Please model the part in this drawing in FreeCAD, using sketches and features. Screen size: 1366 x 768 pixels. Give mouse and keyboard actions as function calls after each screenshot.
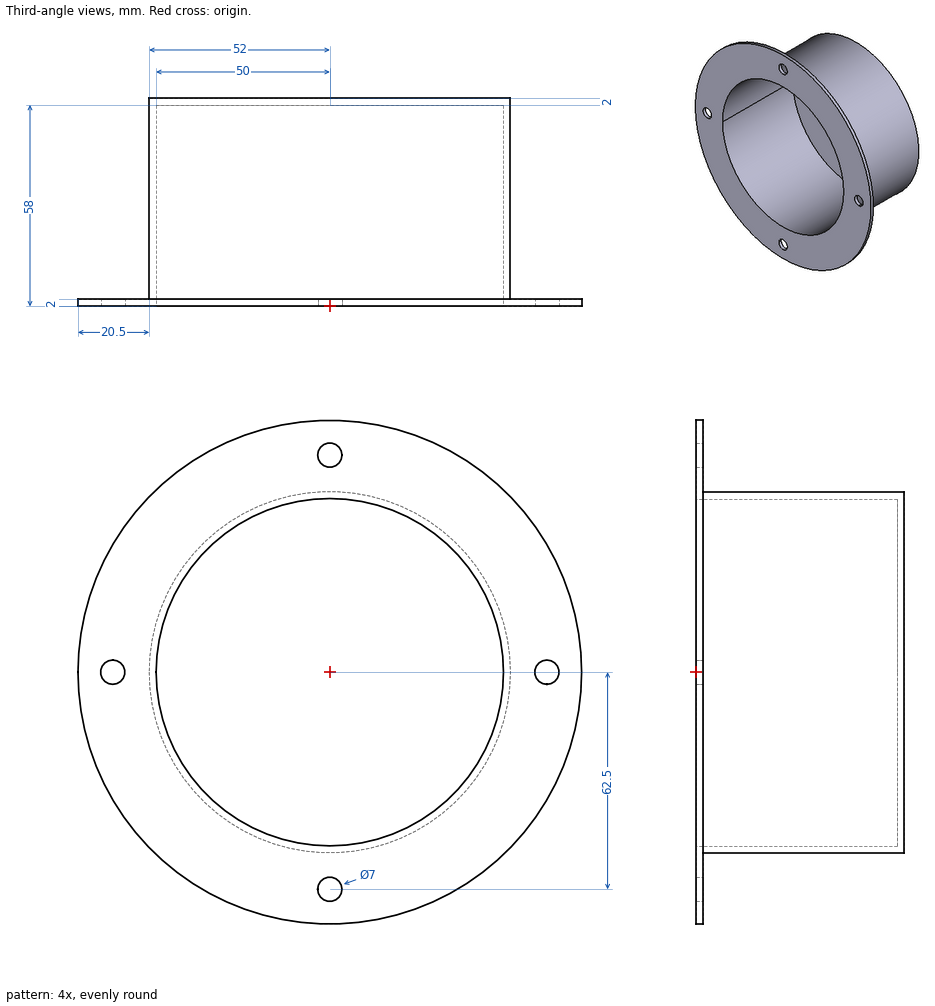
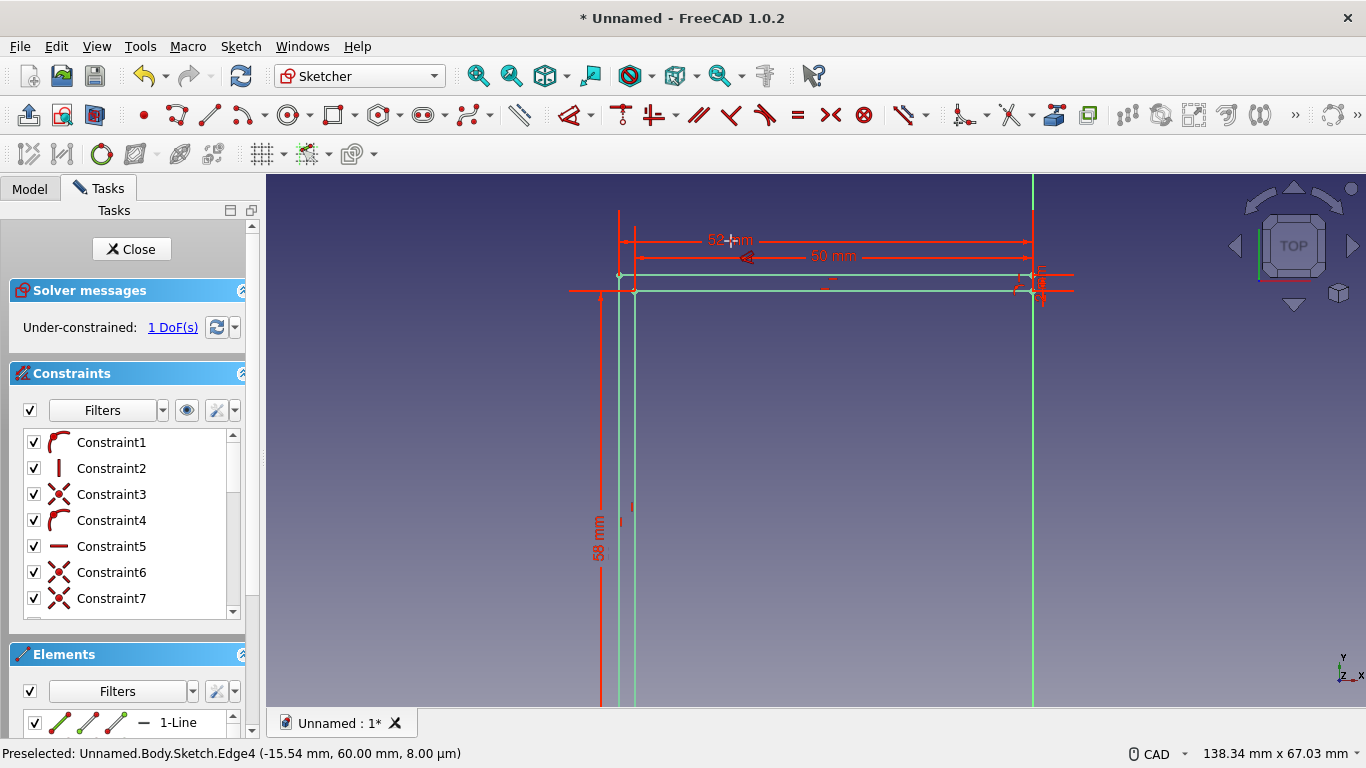
scroll(754, 291, down, 2)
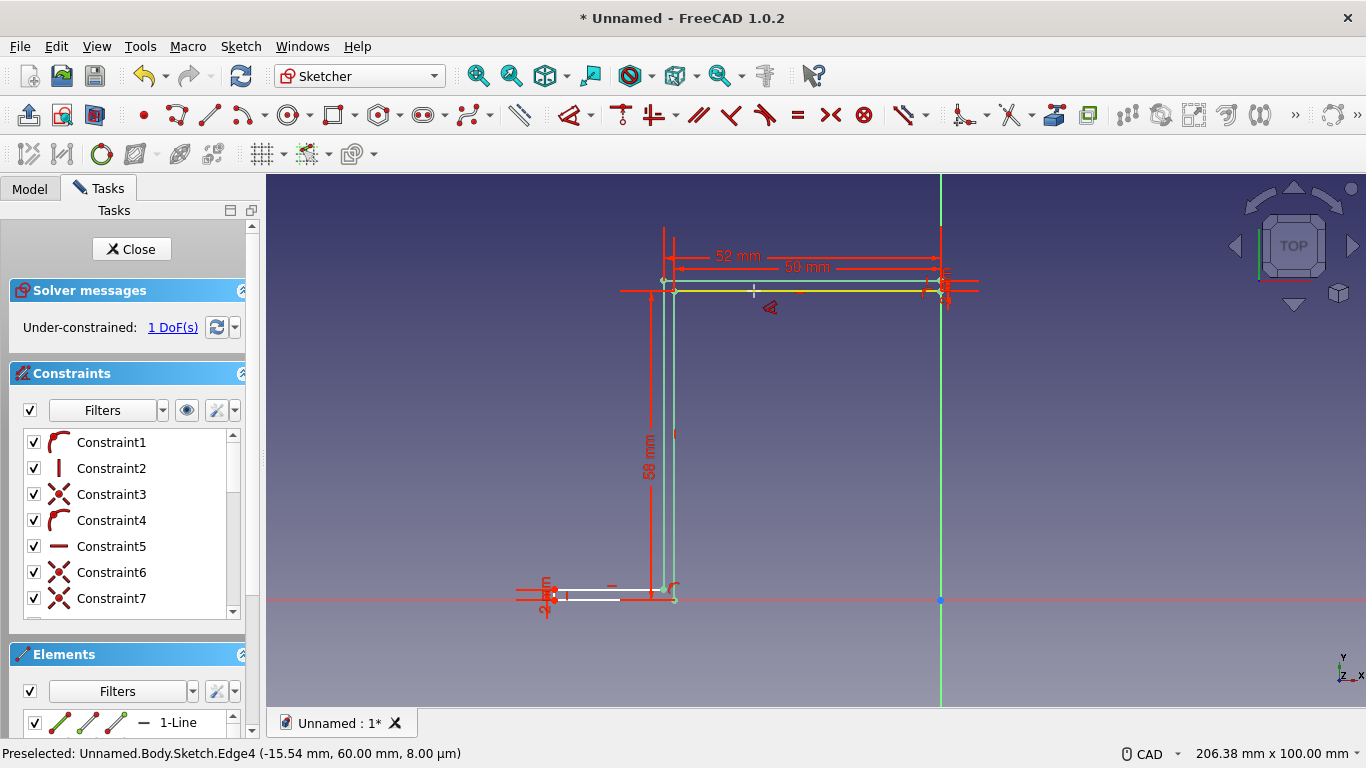
scroll(631, 590, up, 2)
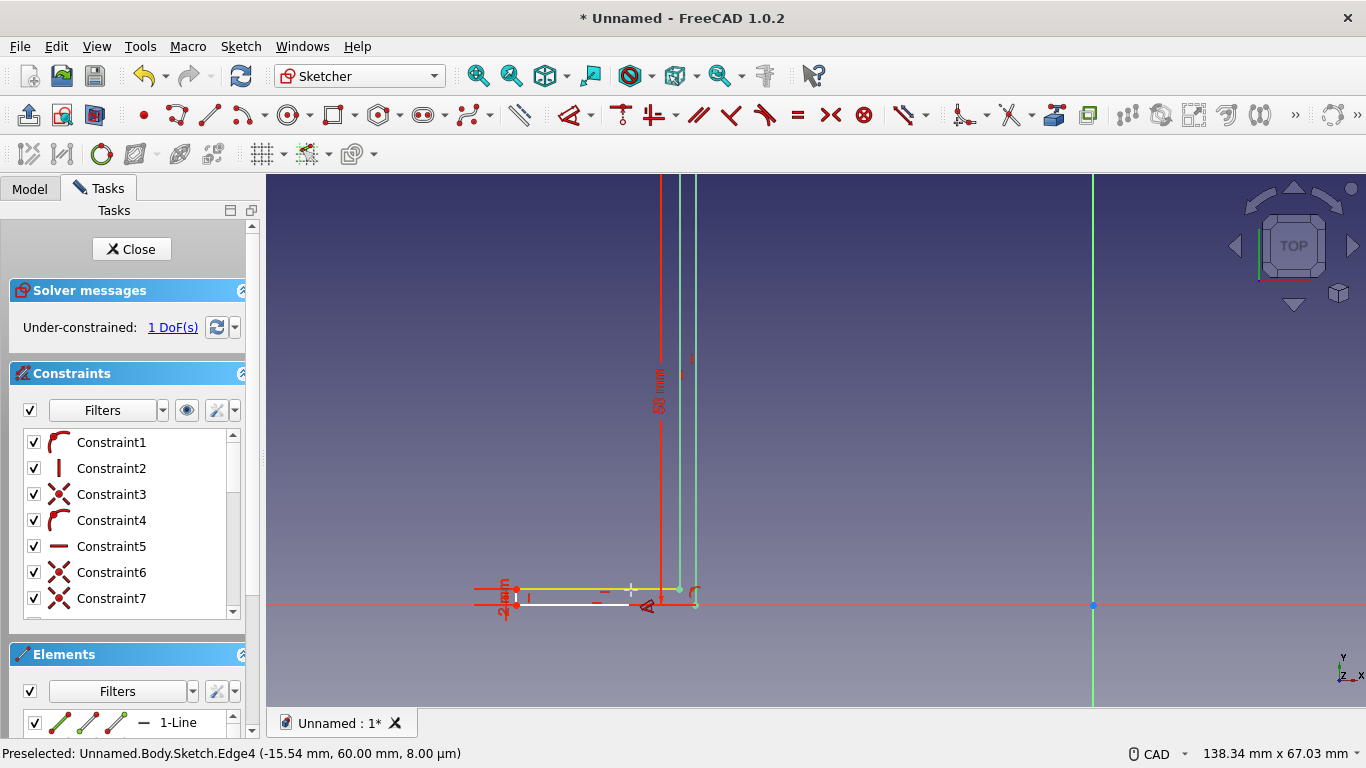
click(631, 589)
click(598, 623)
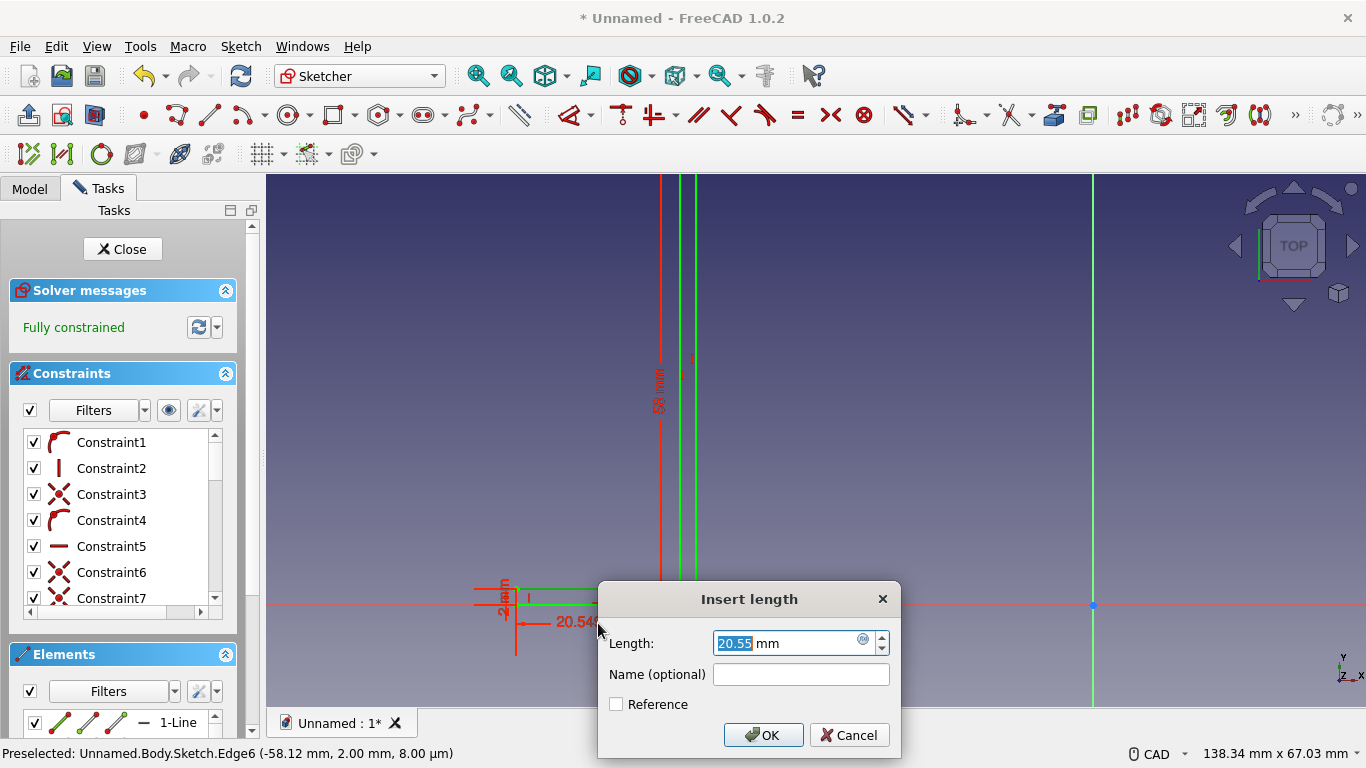
text(20.5)
key(Return)
key(Escape)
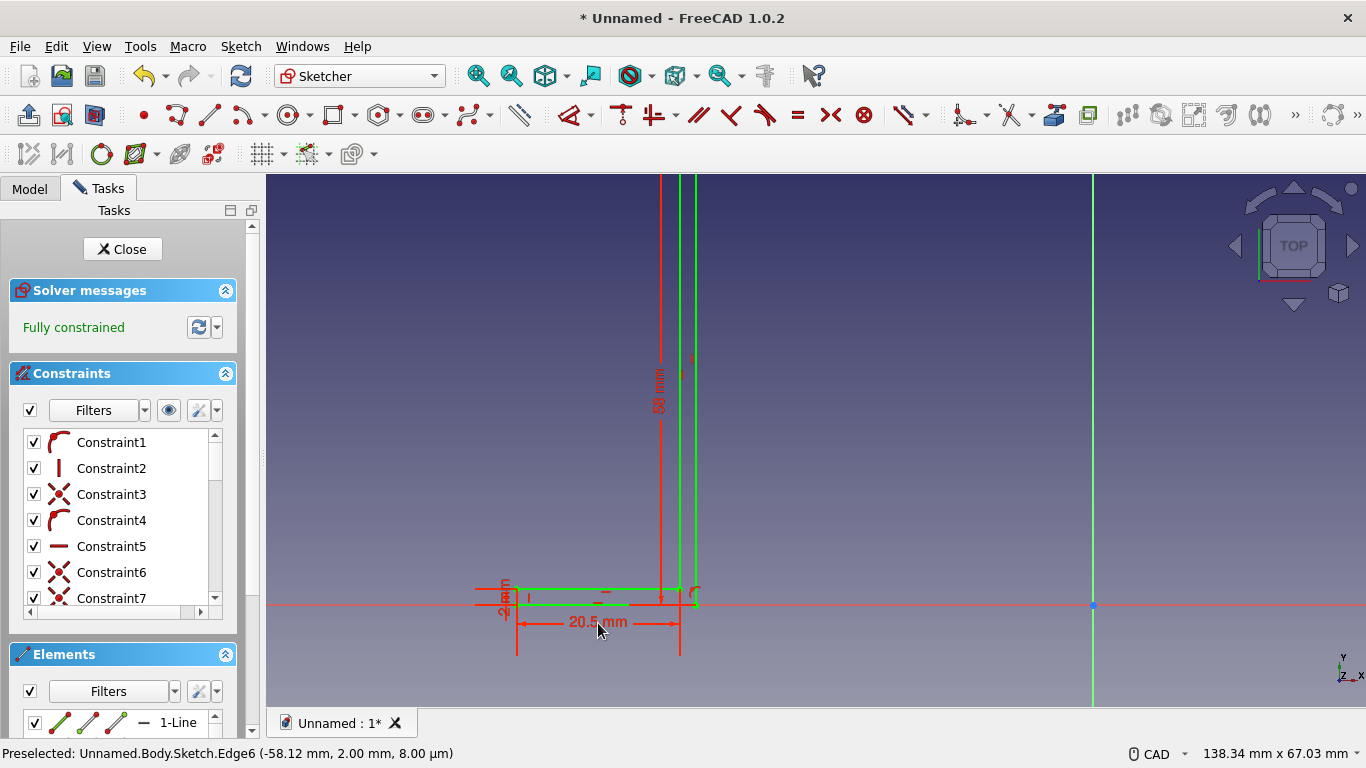
click(123, 249)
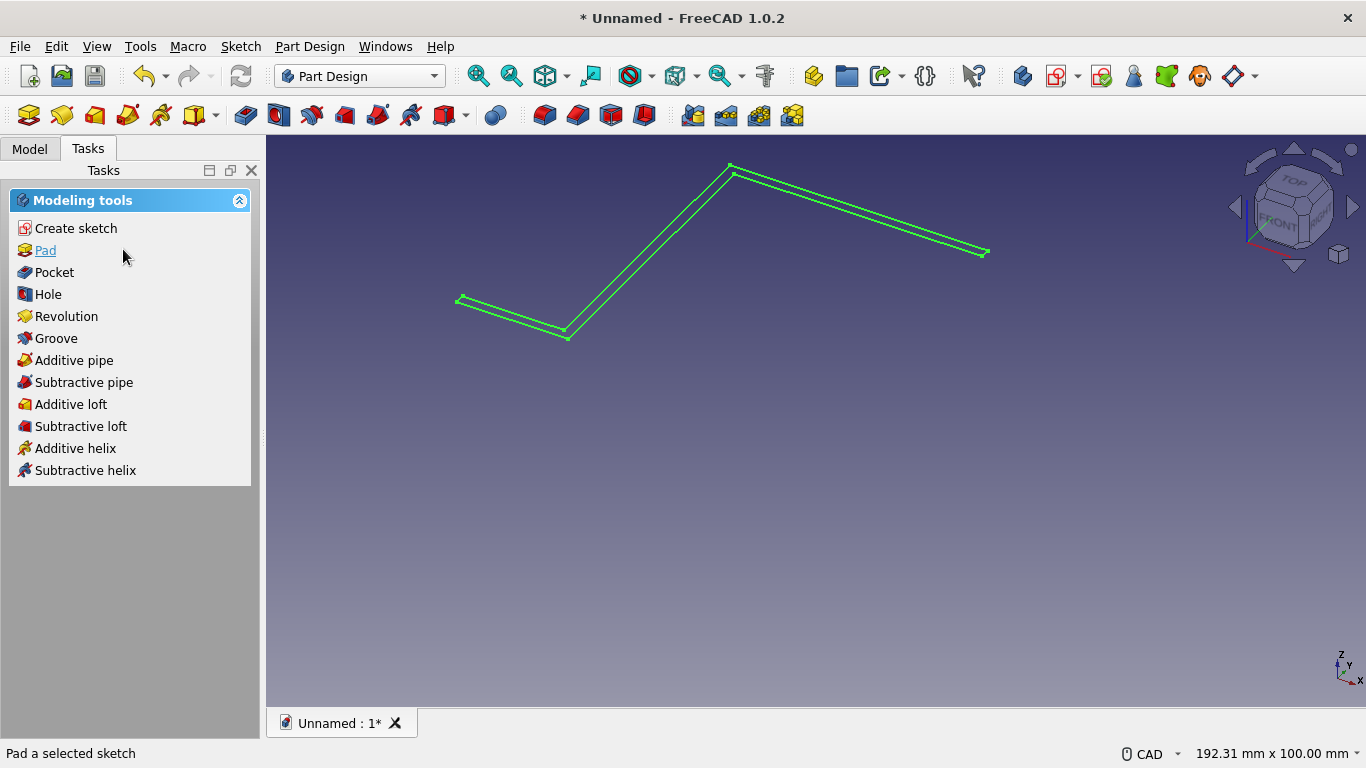
click(62, 116)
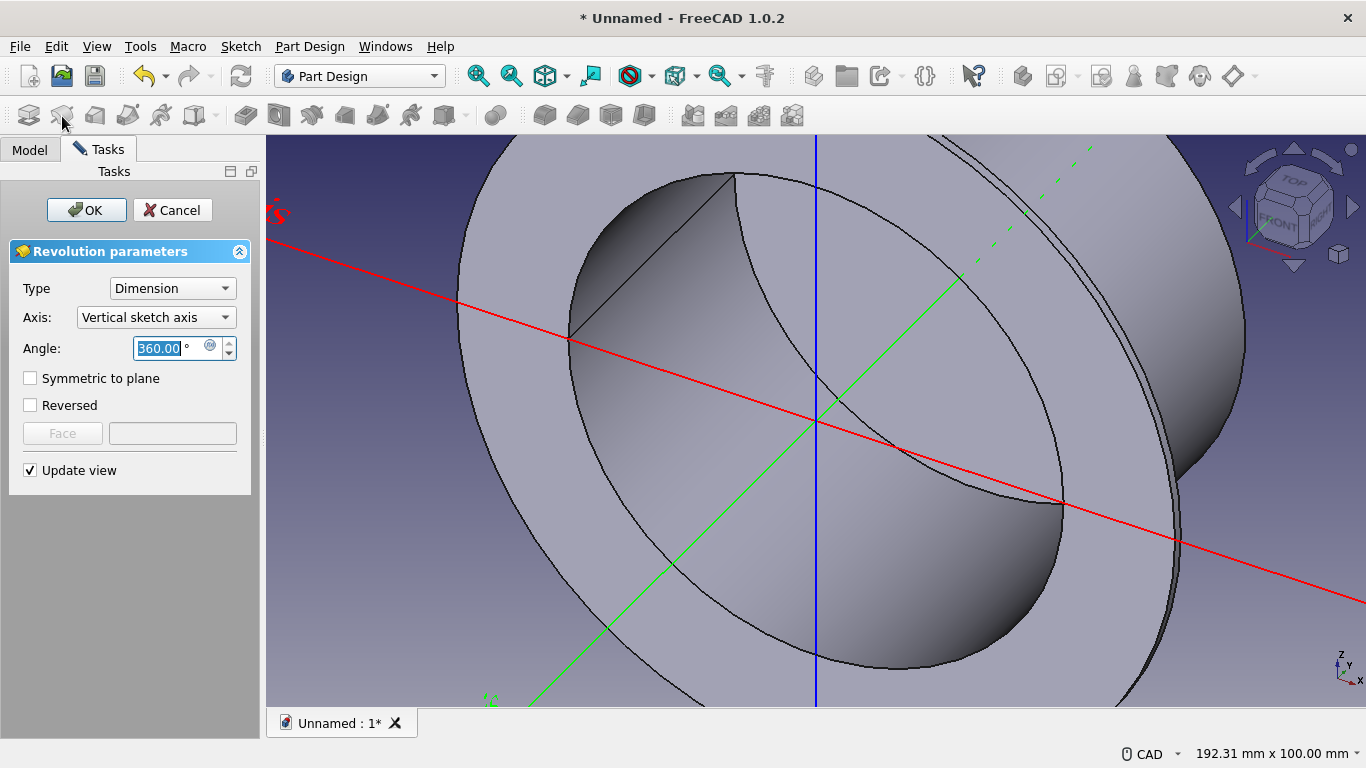
click(87, 210)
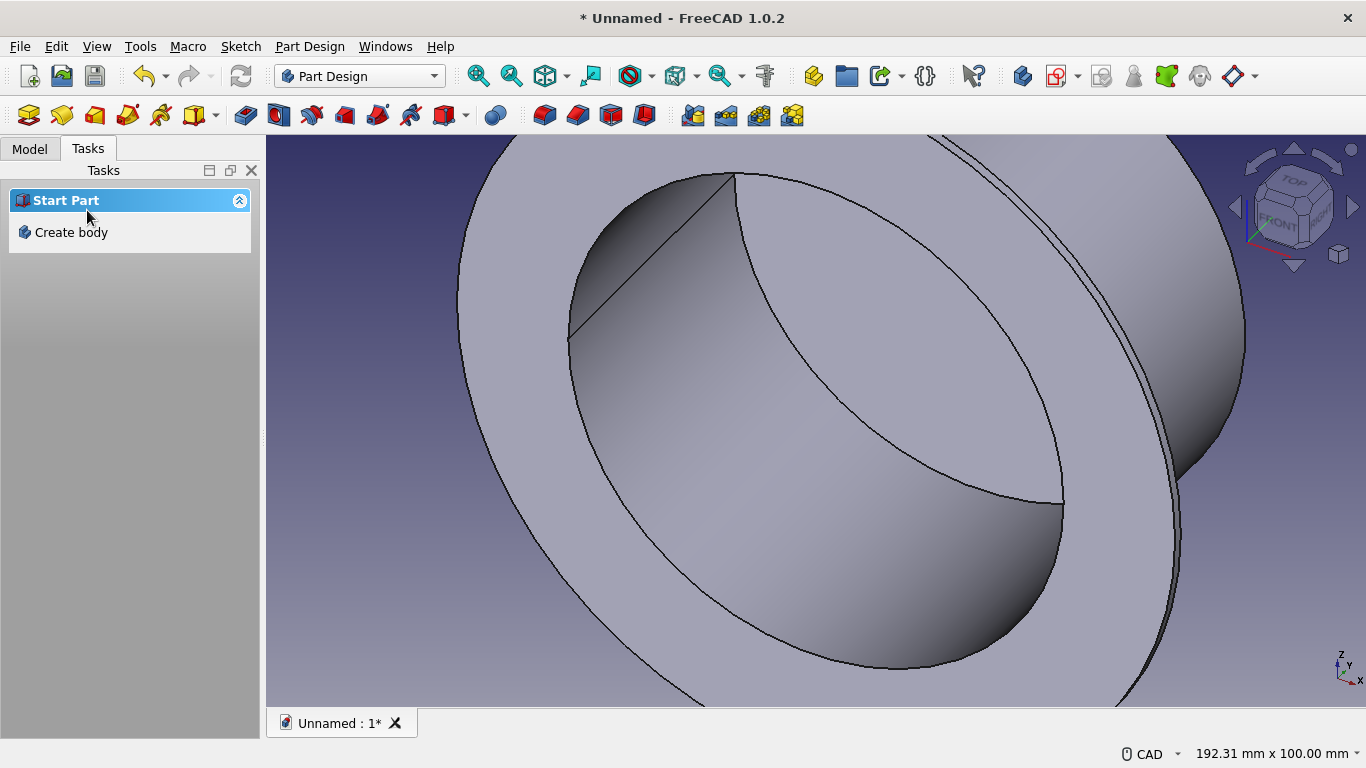
click(479, 76)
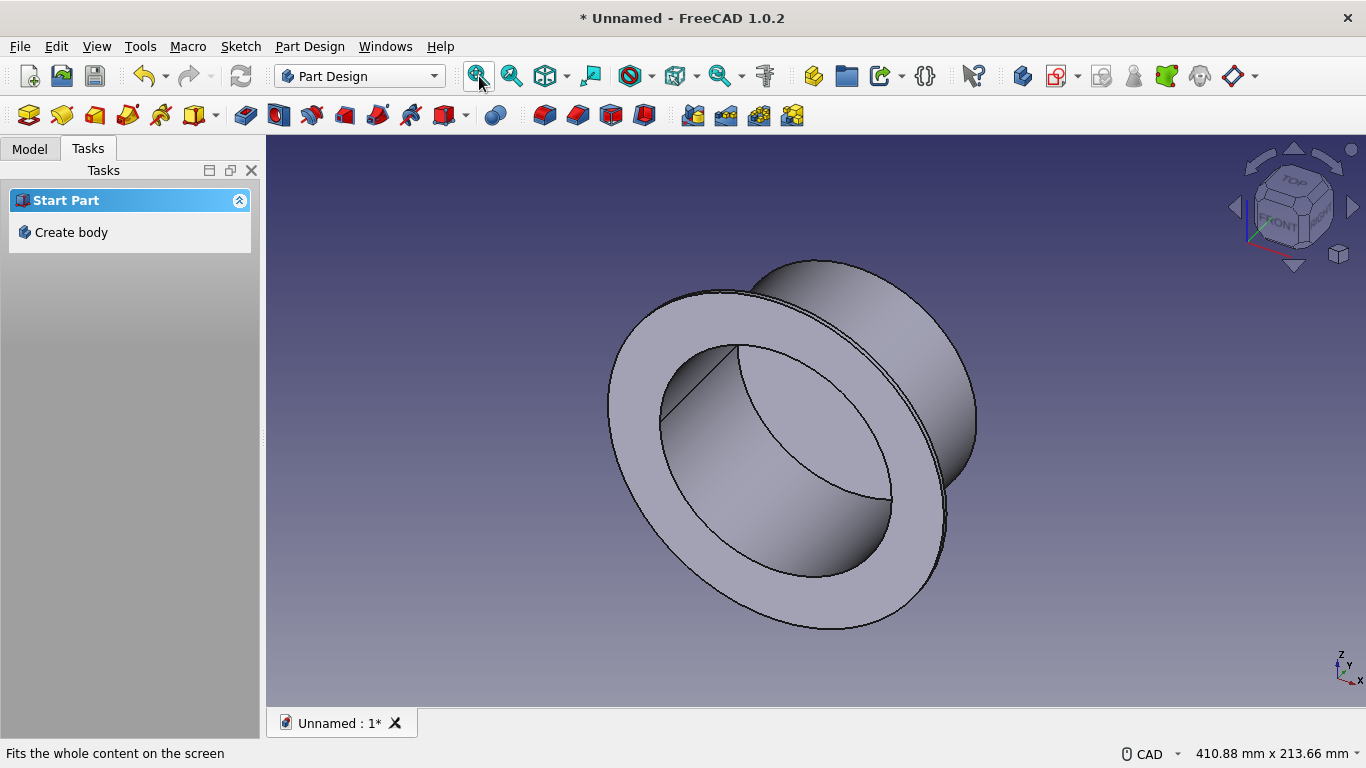
key(4)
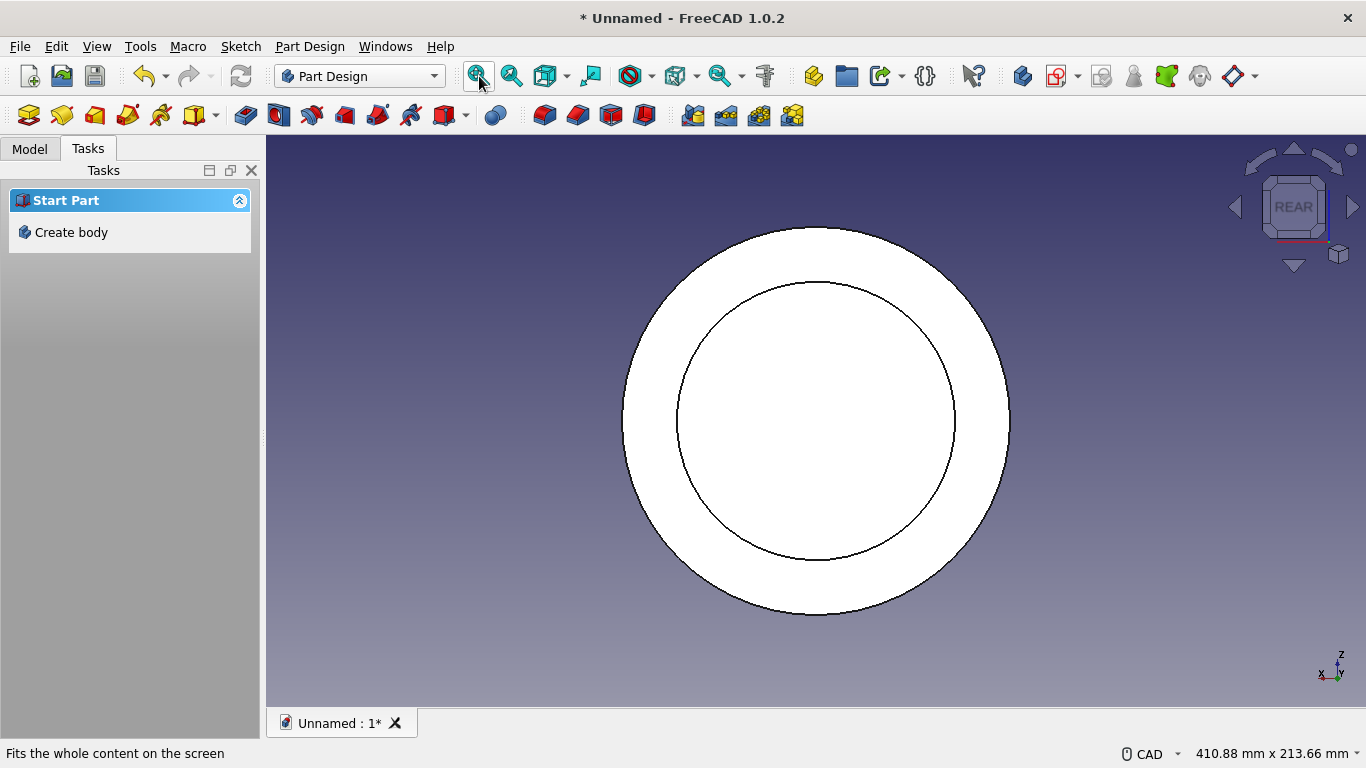
click(650, 420)